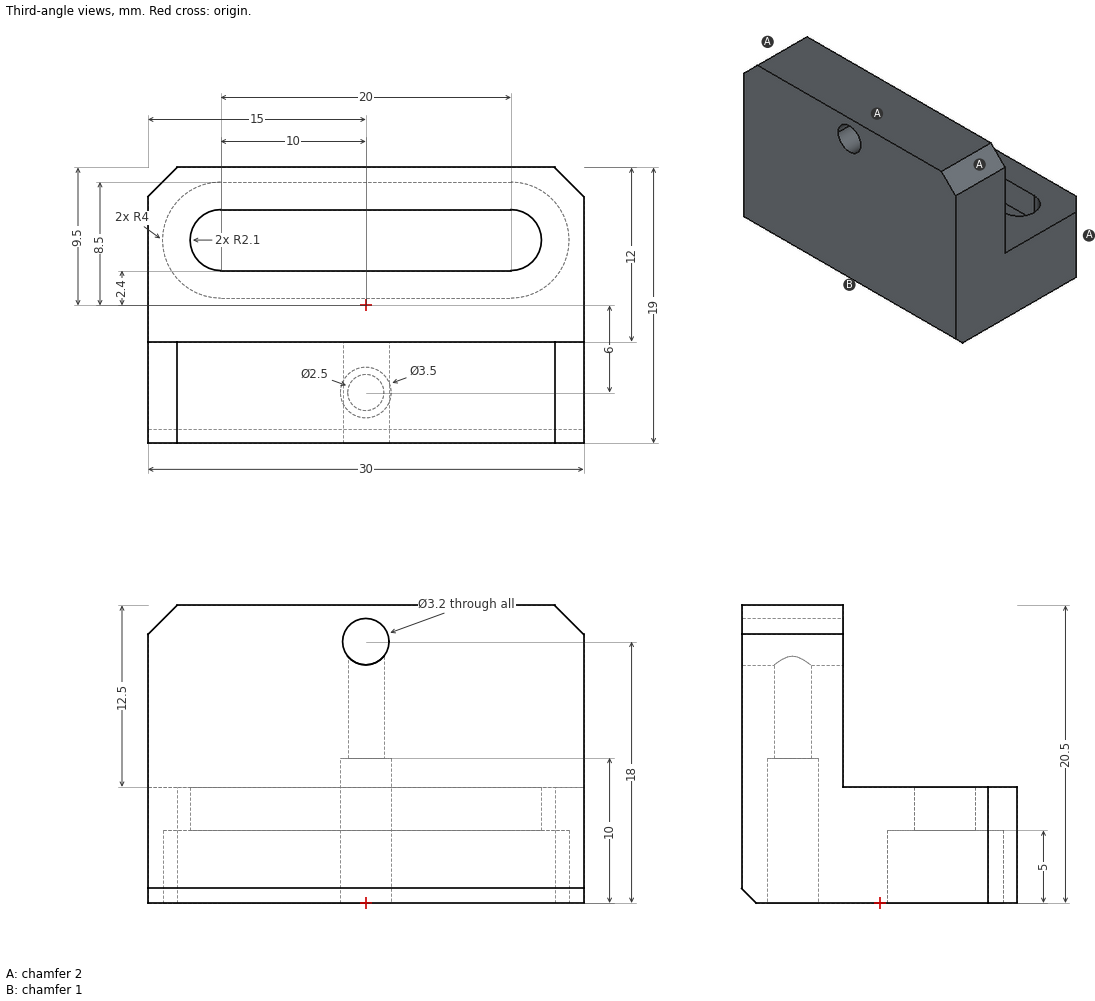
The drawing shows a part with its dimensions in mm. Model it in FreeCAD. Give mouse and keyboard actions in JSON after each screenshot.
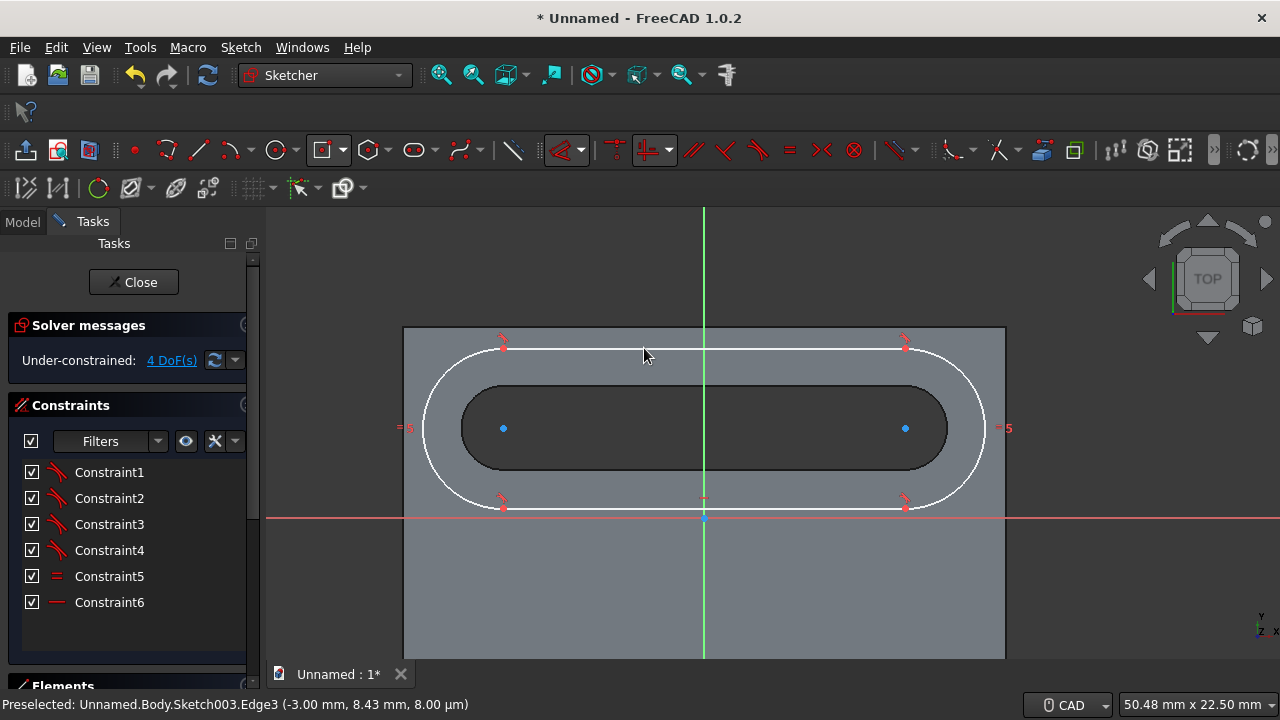
{"action": "left_click", "coordinate": [438, 382]}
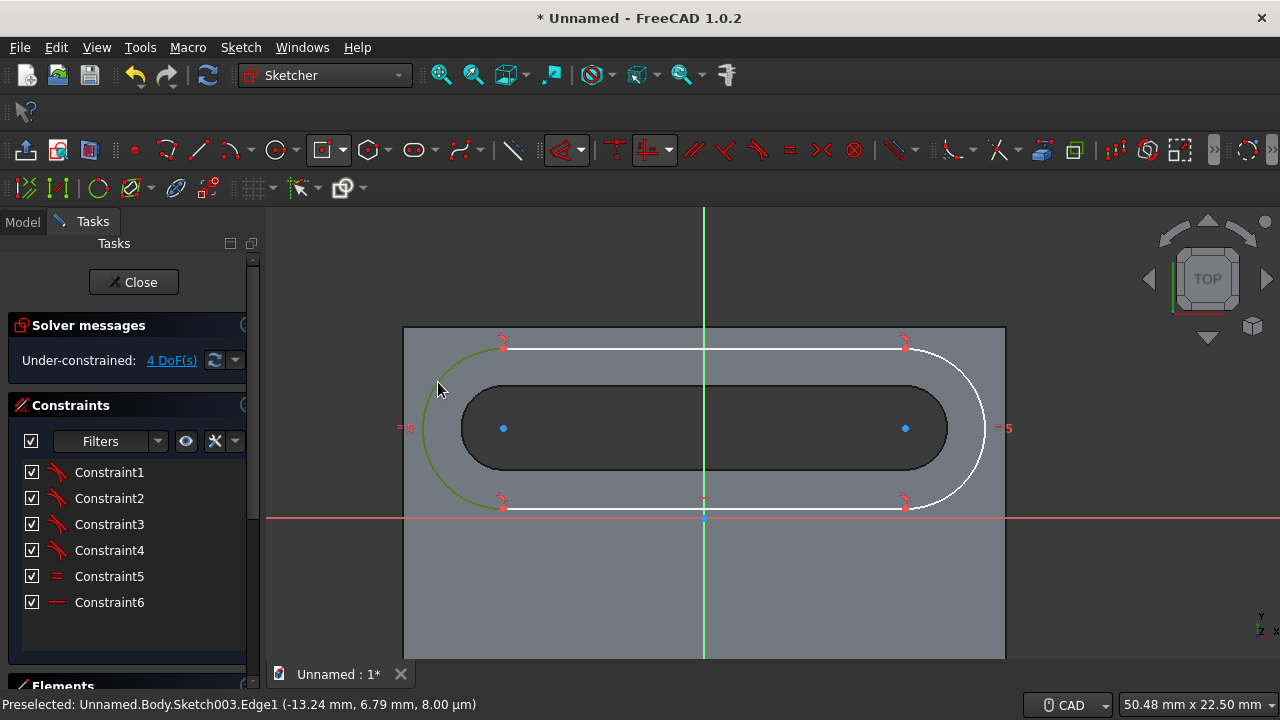
{"action": "left_click", "coordinate": [584, 150]}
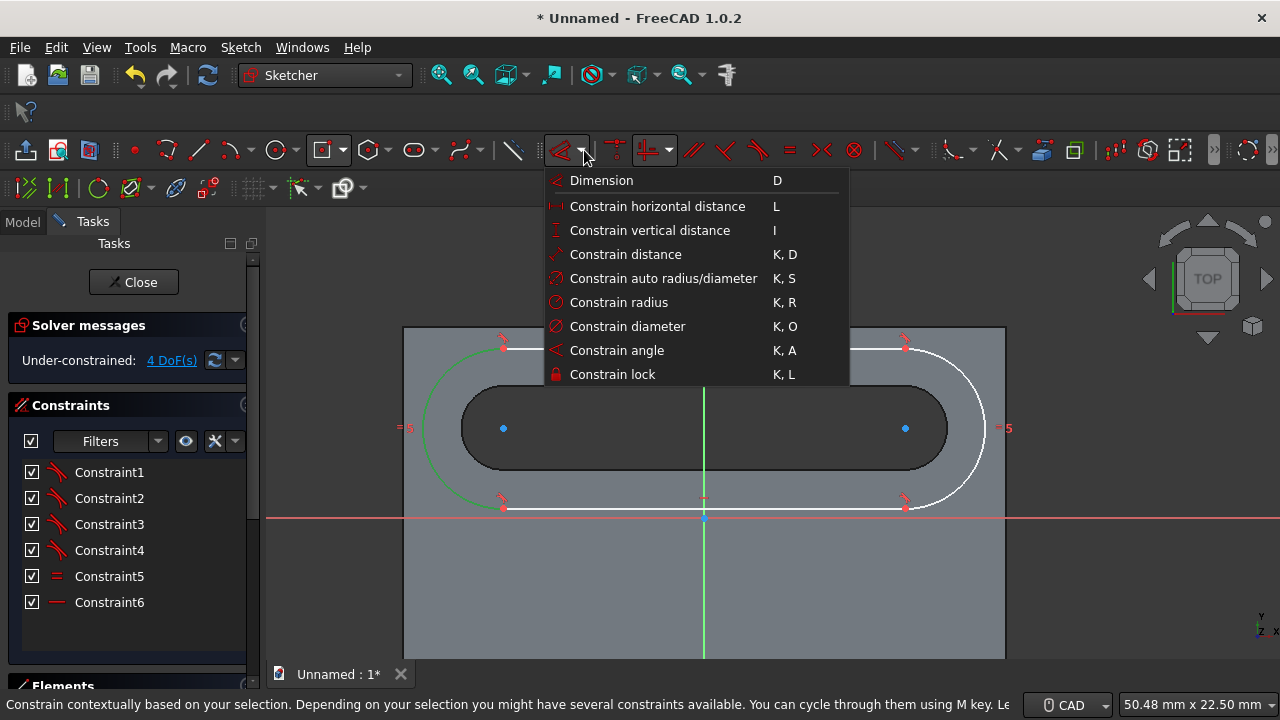
{"action": "left_click", "coordinate": [697, 302]}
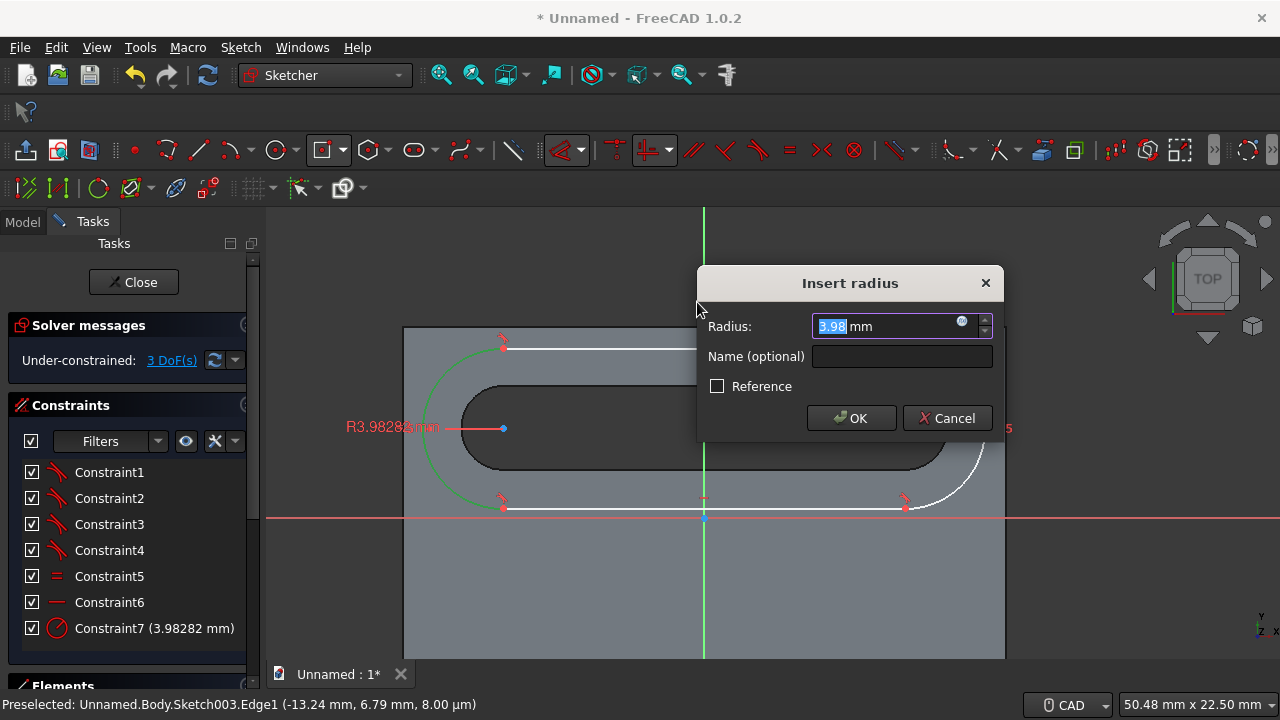
{"action": "type", "text": "4"}
{"action": "key", "text": "Return"}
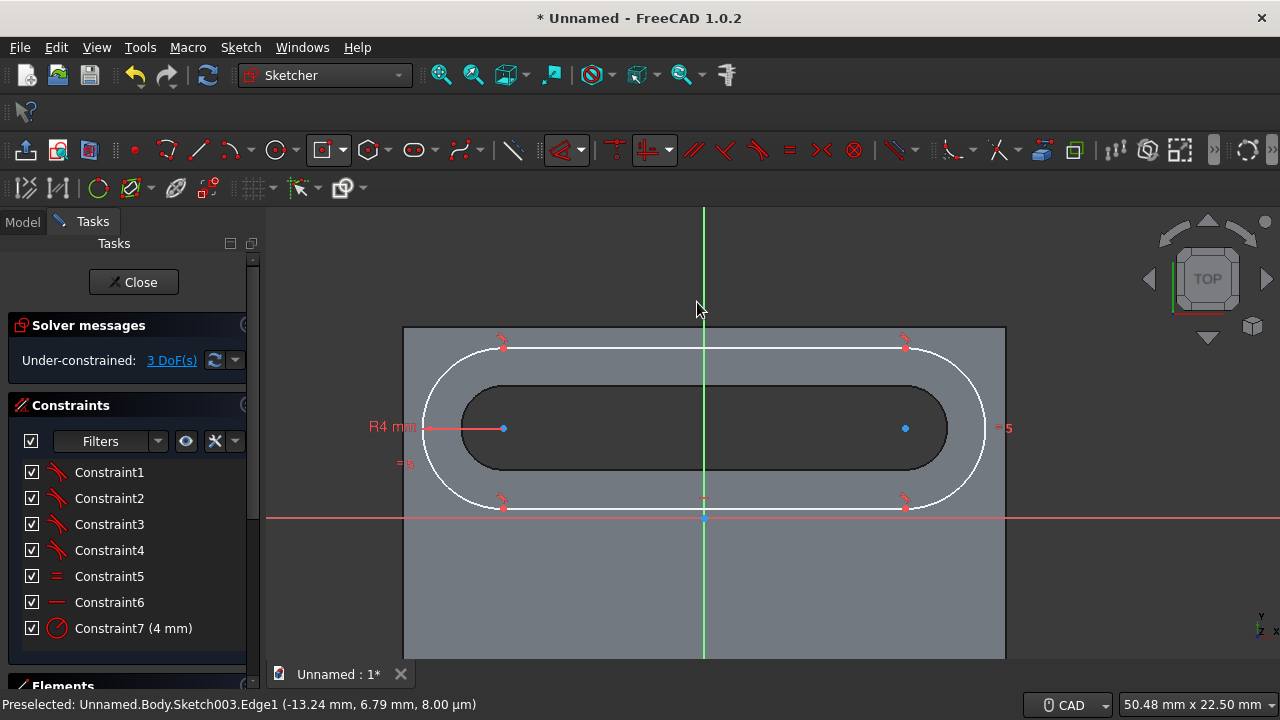
{"action": "left_click", "coordinate": [624, 348]}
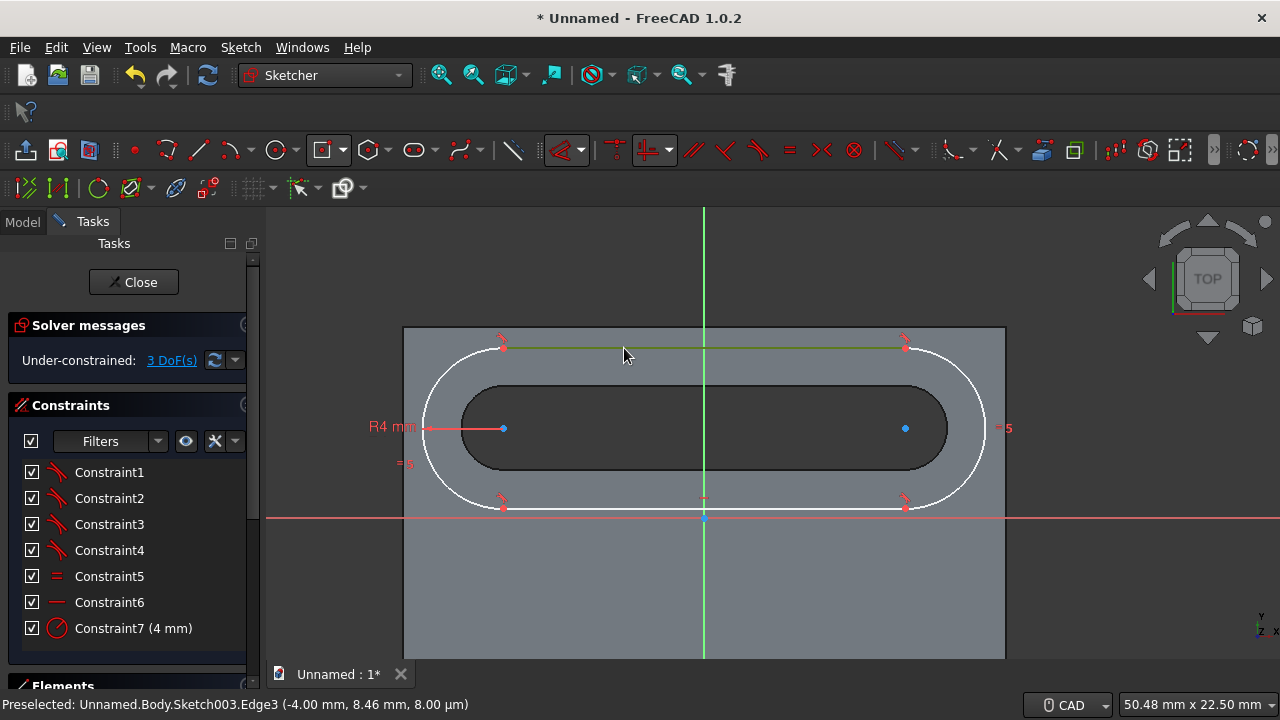
{"action": "key", "text": "l"}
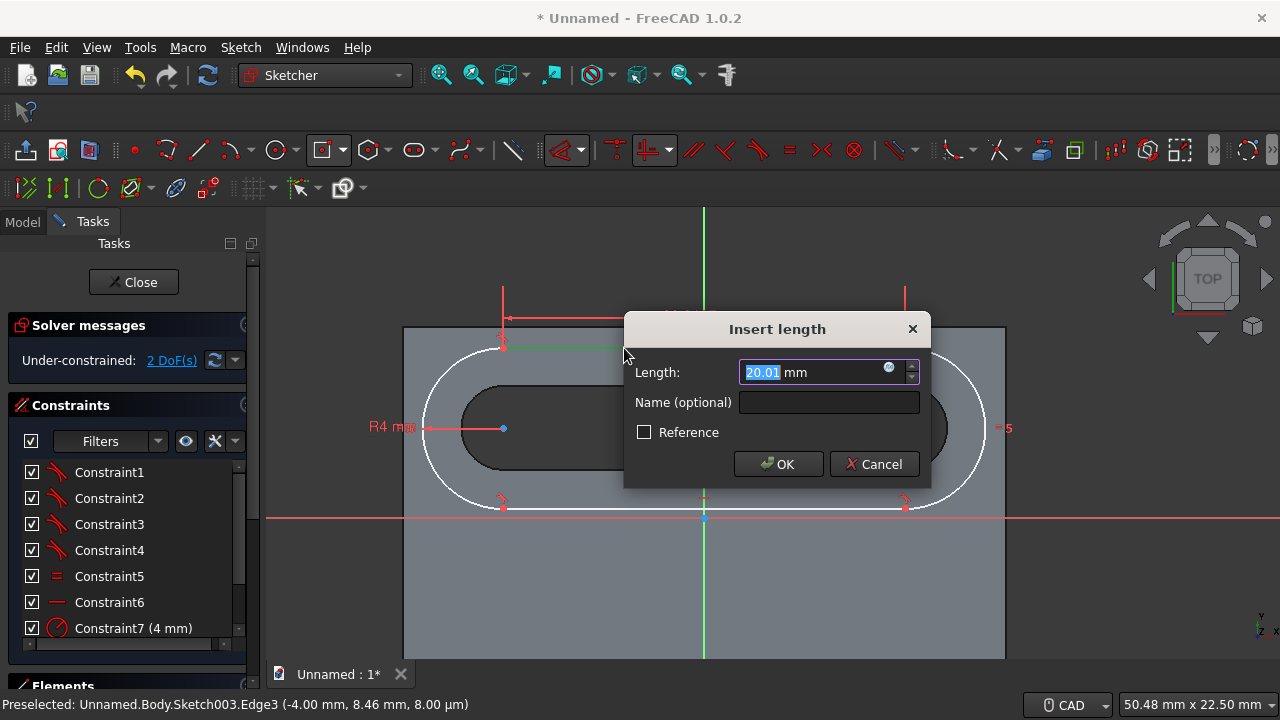
{"action": "type", "text": "20"}
{"action": "key", "text": "Return"}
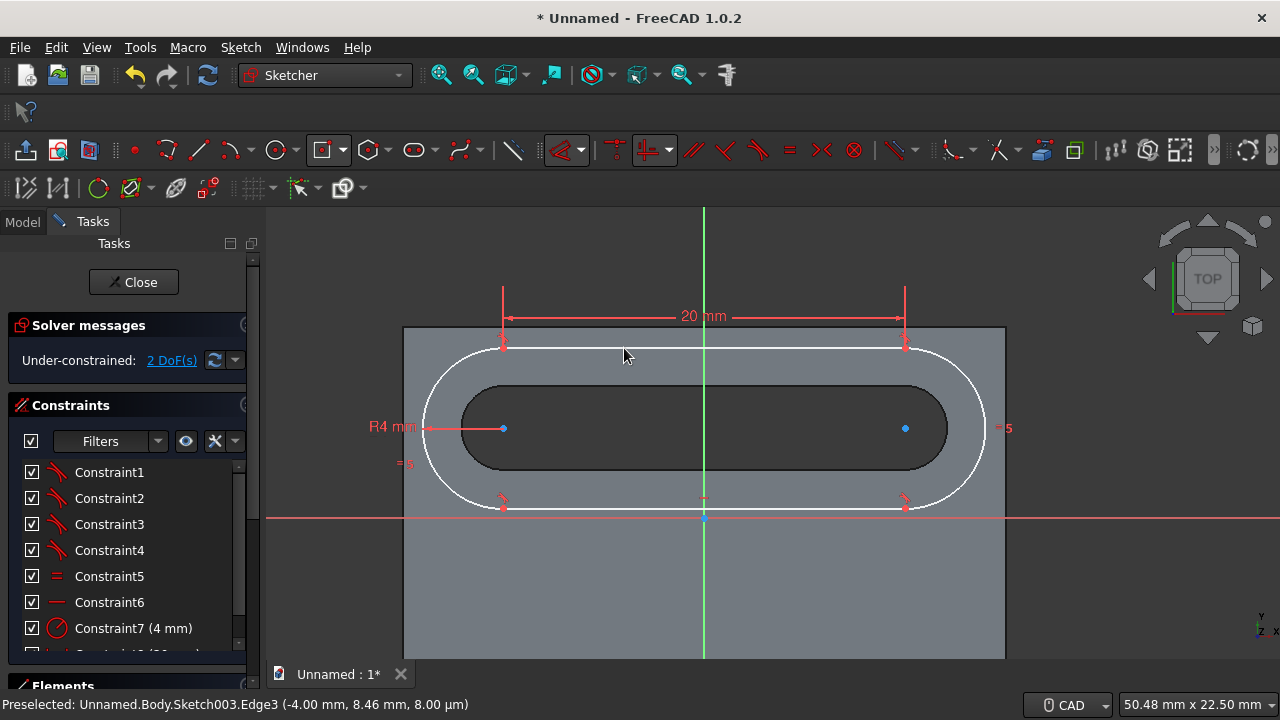
{"action": "left_click", "coordinate": [503, 348]}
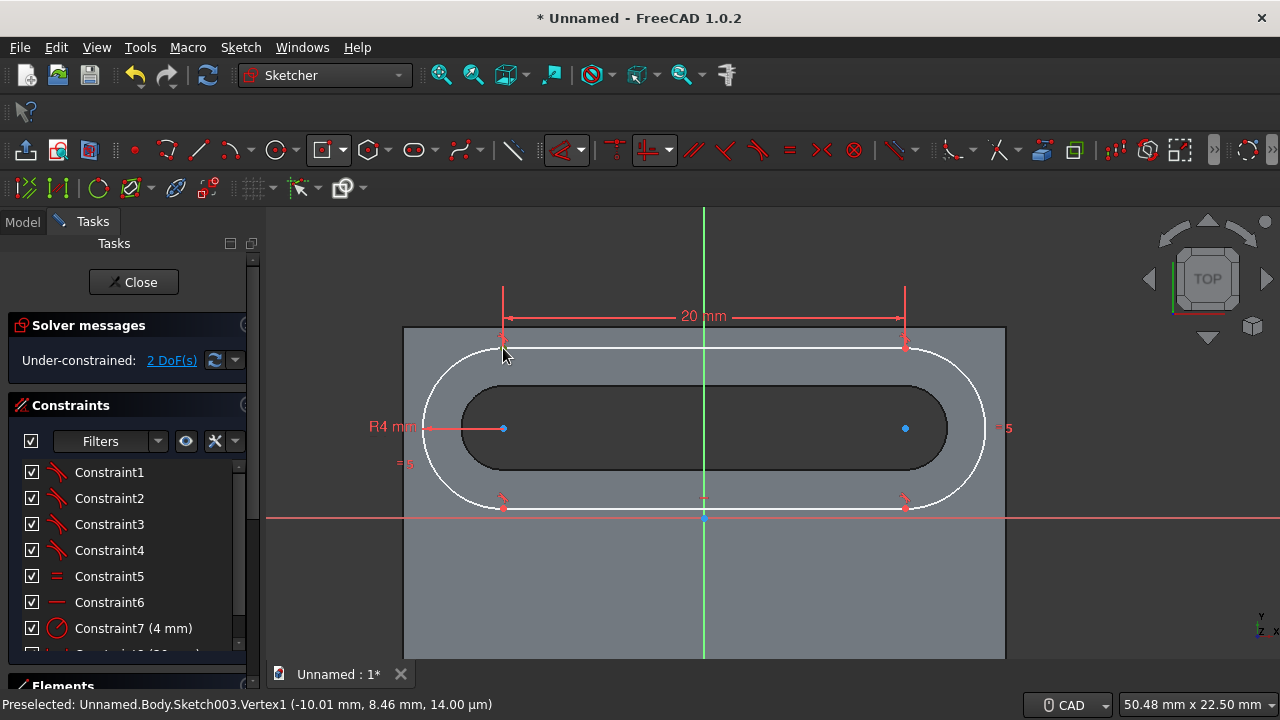
{"action": "key", "text": "l"}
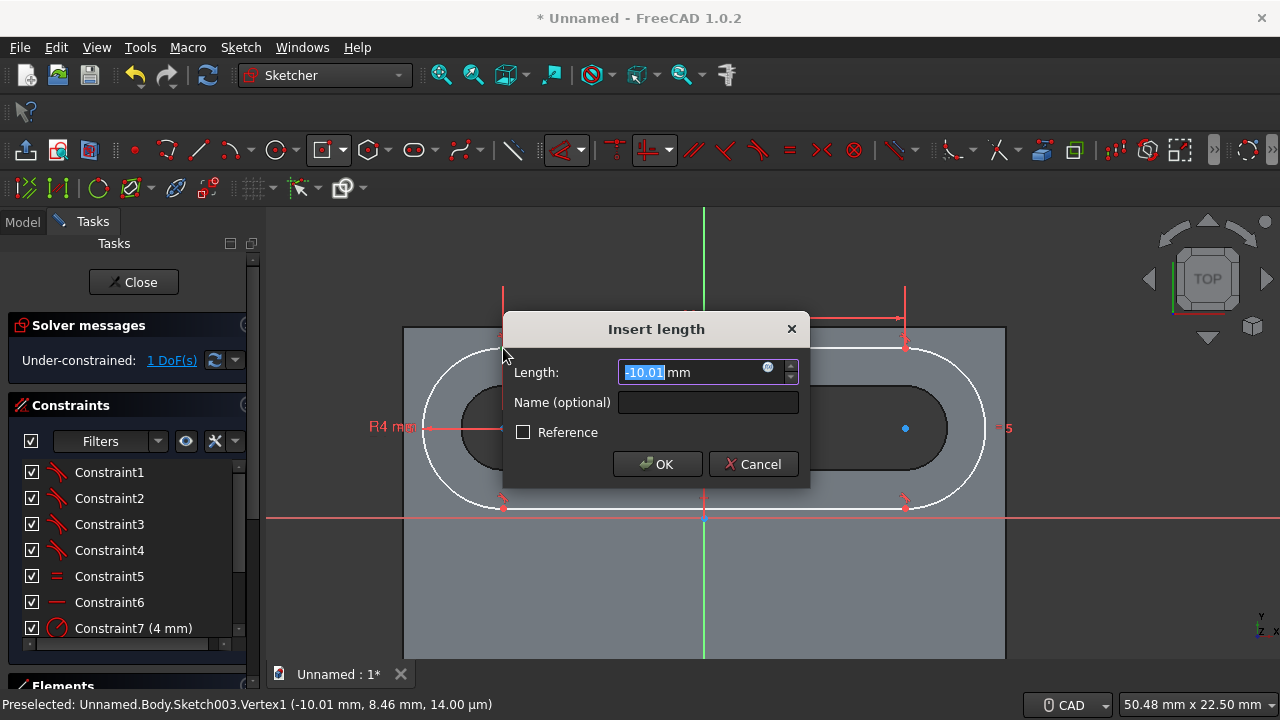
{"action": "type", "text": "-10"}
{"action": "key", "text": "Return"}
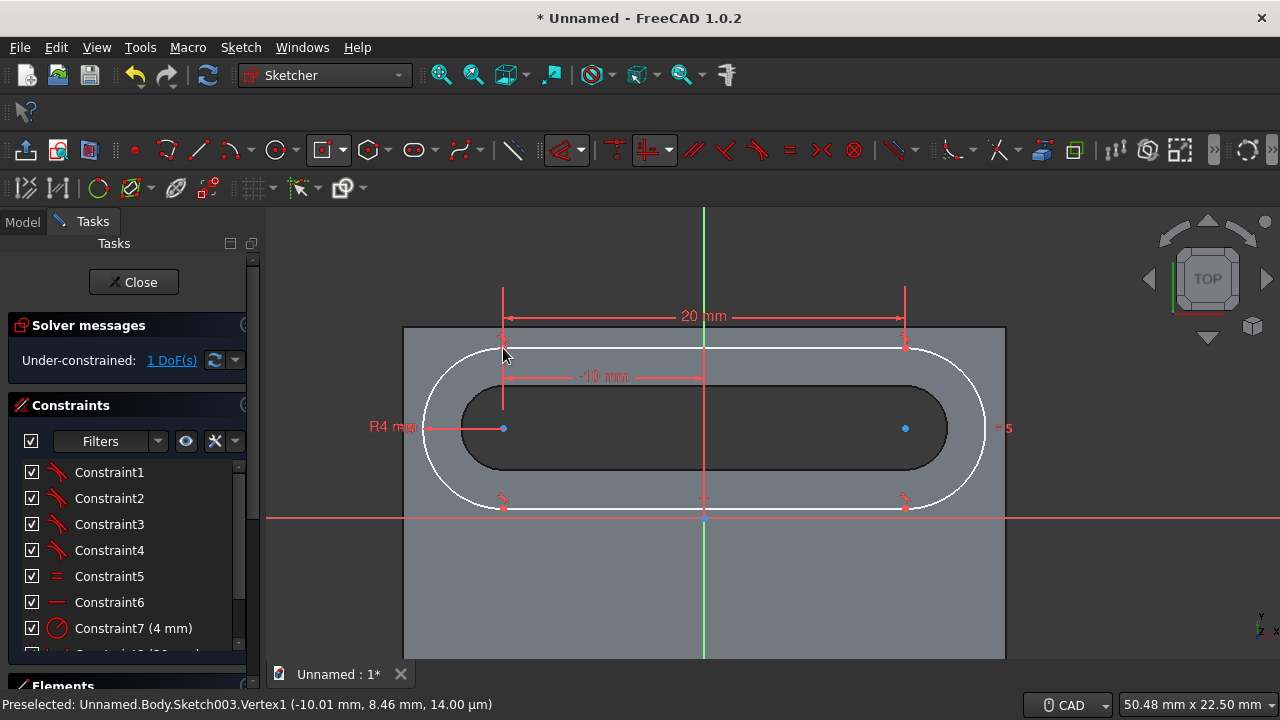
{"action": "left_click", "coordinate": [503, 348]}